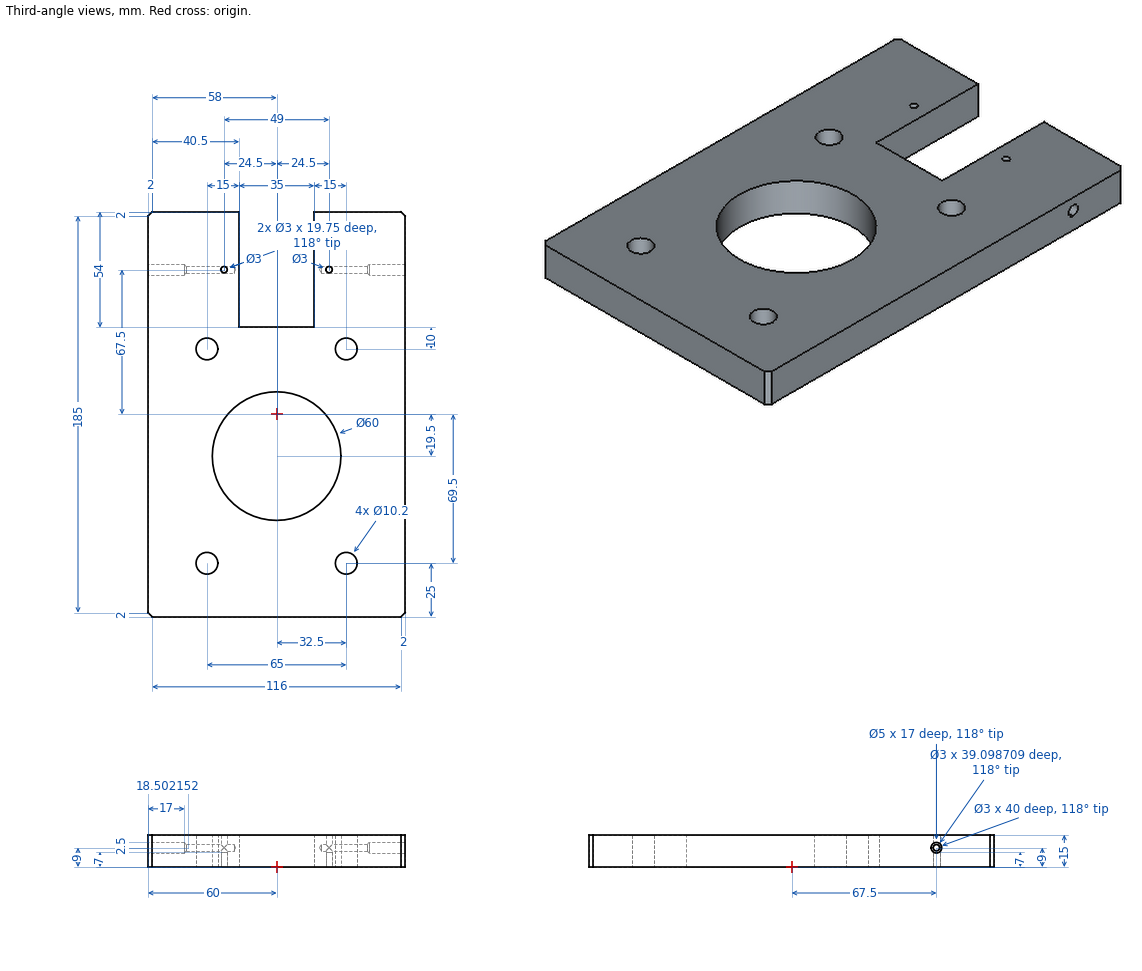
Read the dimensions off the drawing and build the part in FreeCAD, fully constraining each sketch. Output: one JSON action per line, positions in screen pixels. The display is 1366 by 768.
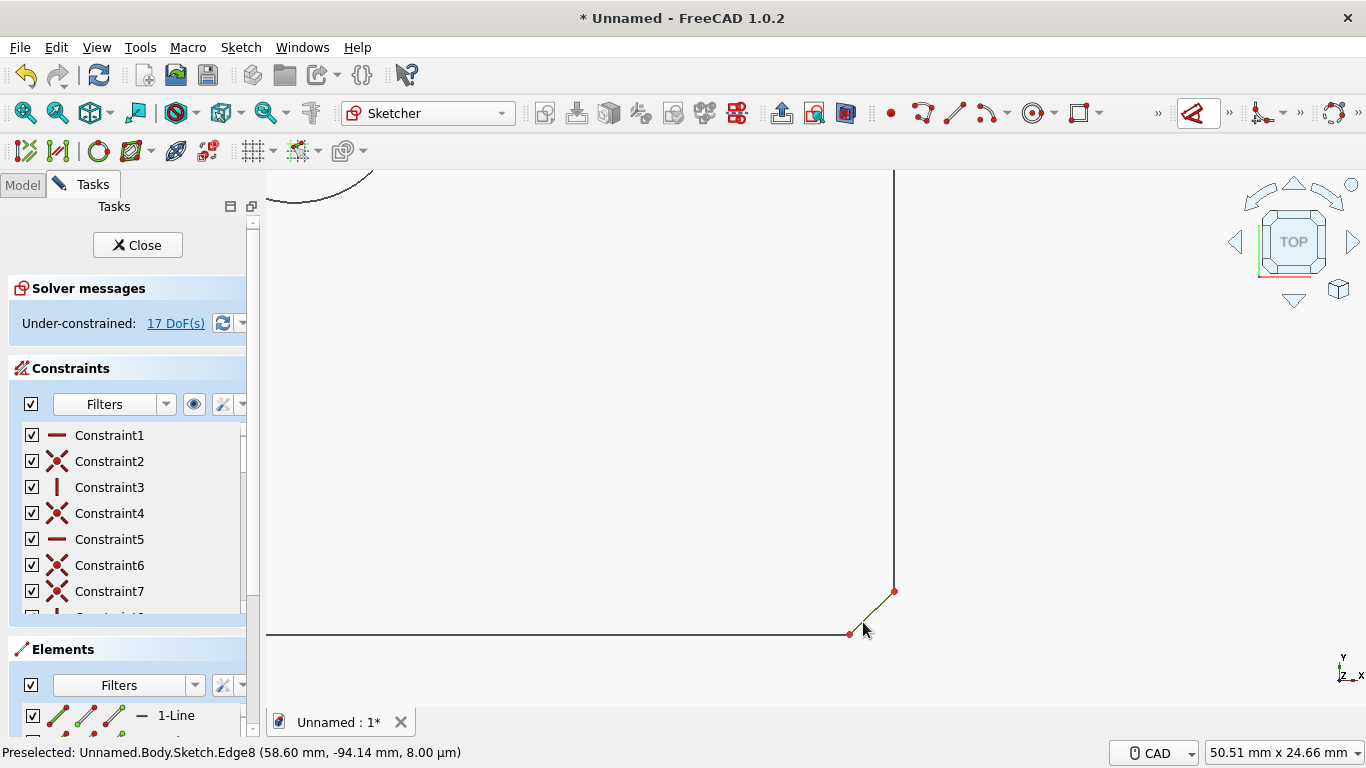
{"action": "key", "text": "l"}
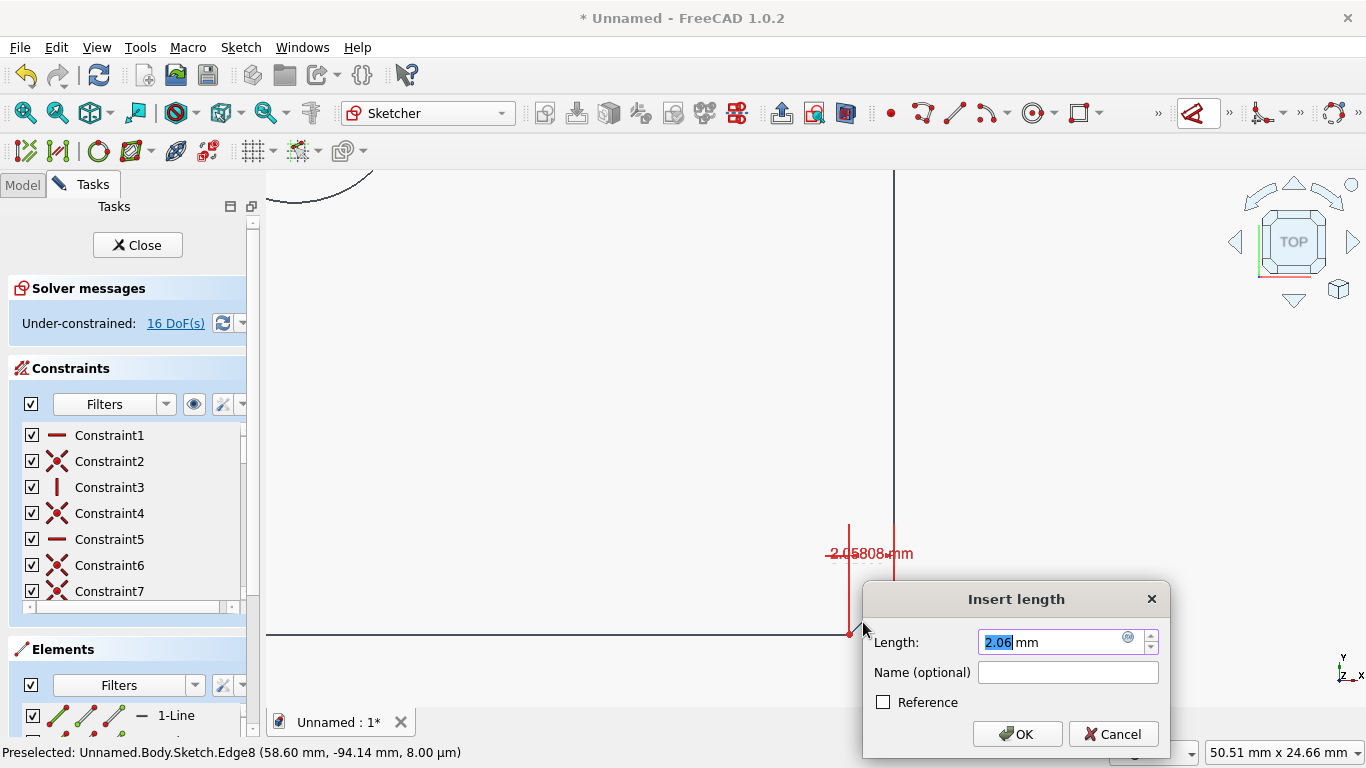
{"action": "type", "text": "2"}
{"action": "key", "text": "Return"}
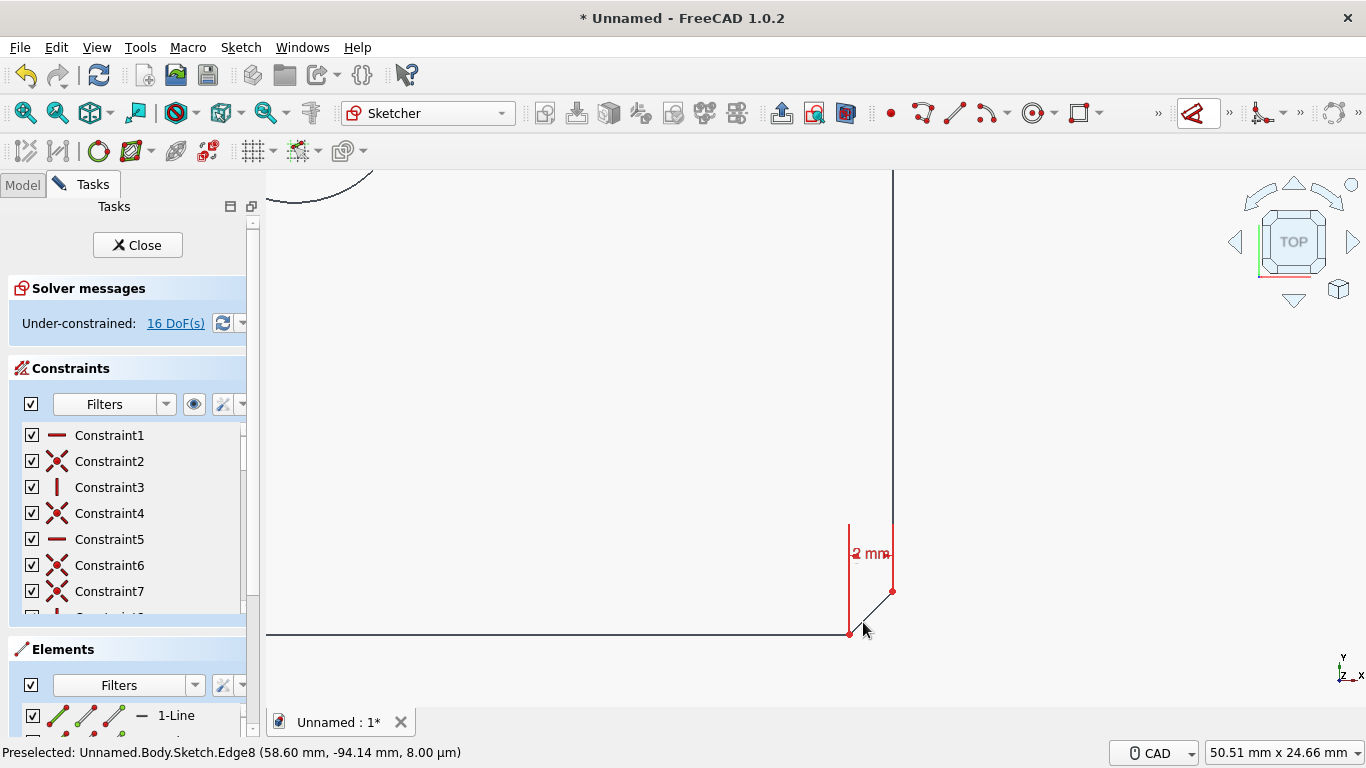
{"action": "left_click", "coordinate": [862, 622]}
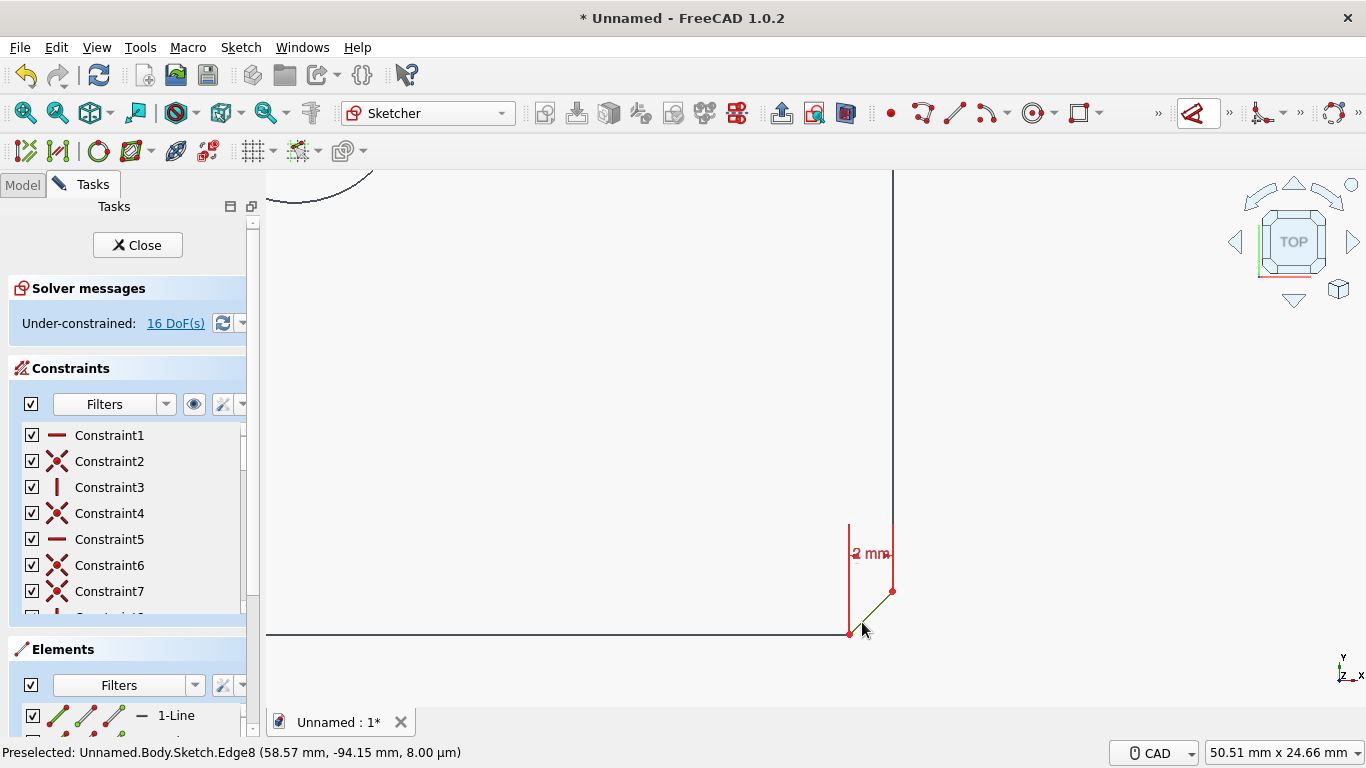
{"action": "key", "text": "i"}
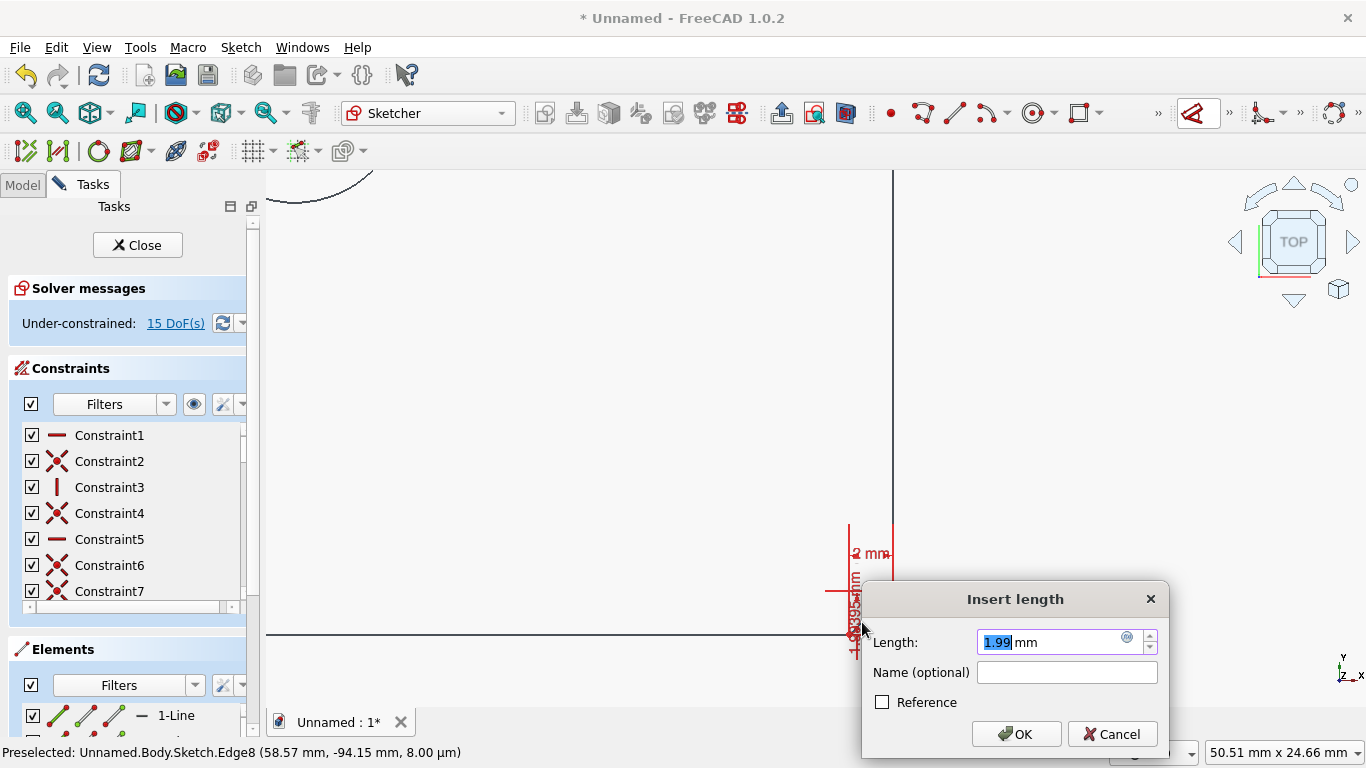
{"action": "type", "text": "2"}
{"action": "key", "text": "Return"}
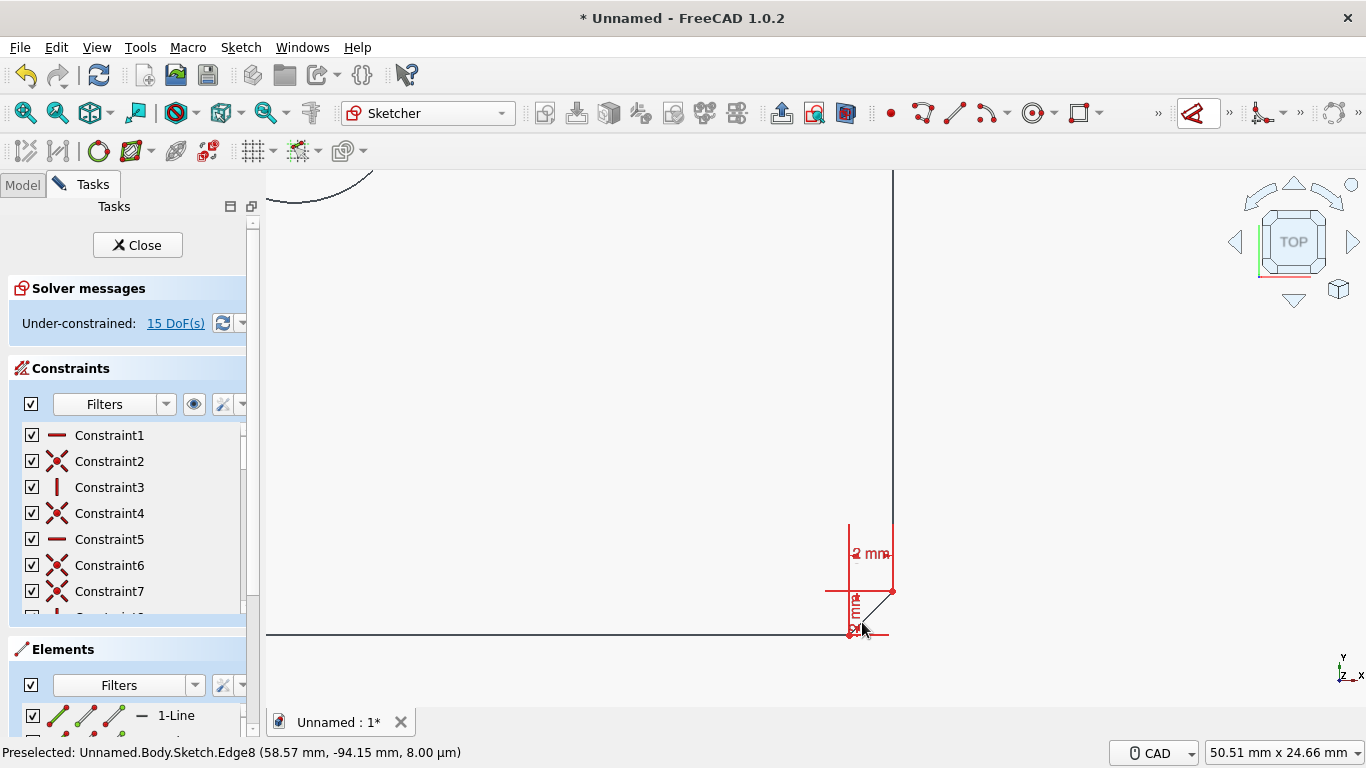
{"action": "scroll", "coordinate": [863, 625], "scroll_direction": "down", "scroll_amount": 12}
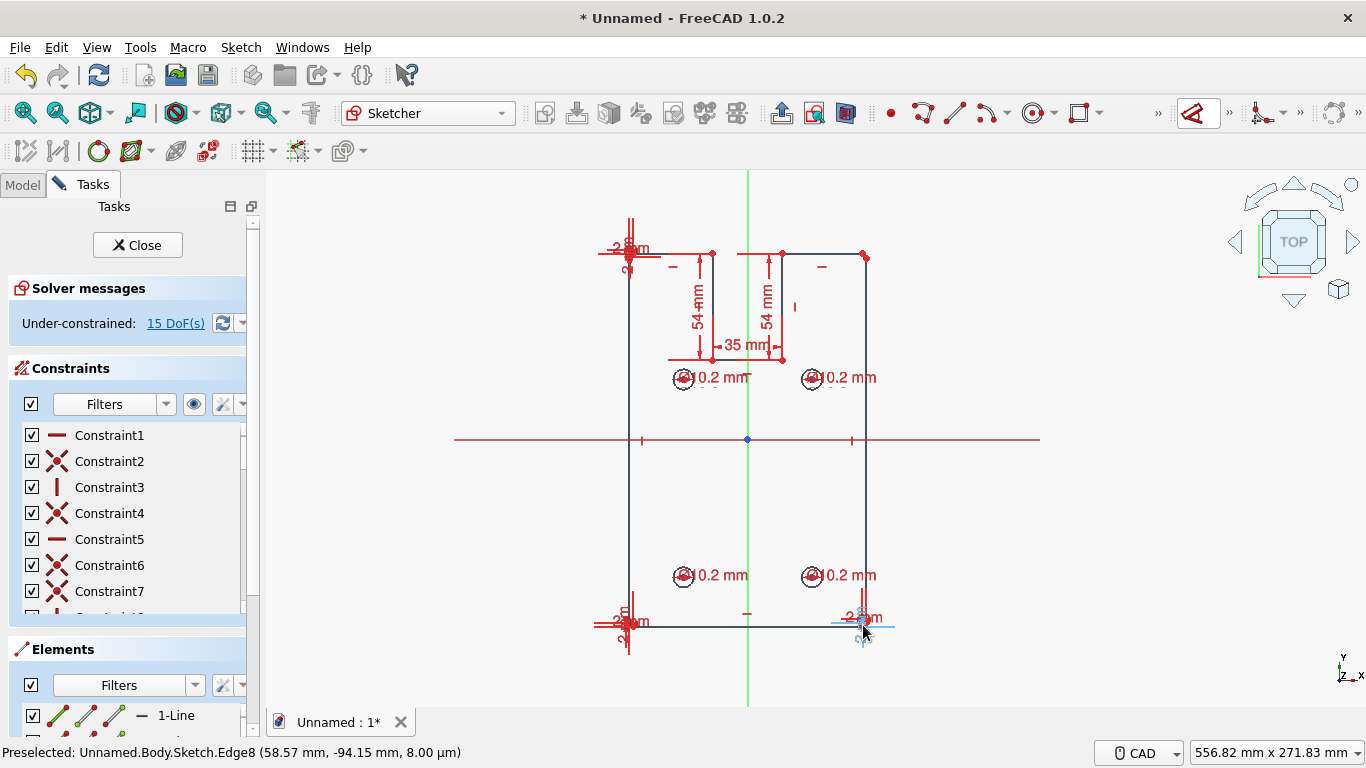
{"action": "scroll", "coordinate": [865, 257], "scroll_direction": "up", "scroll_amount": 12}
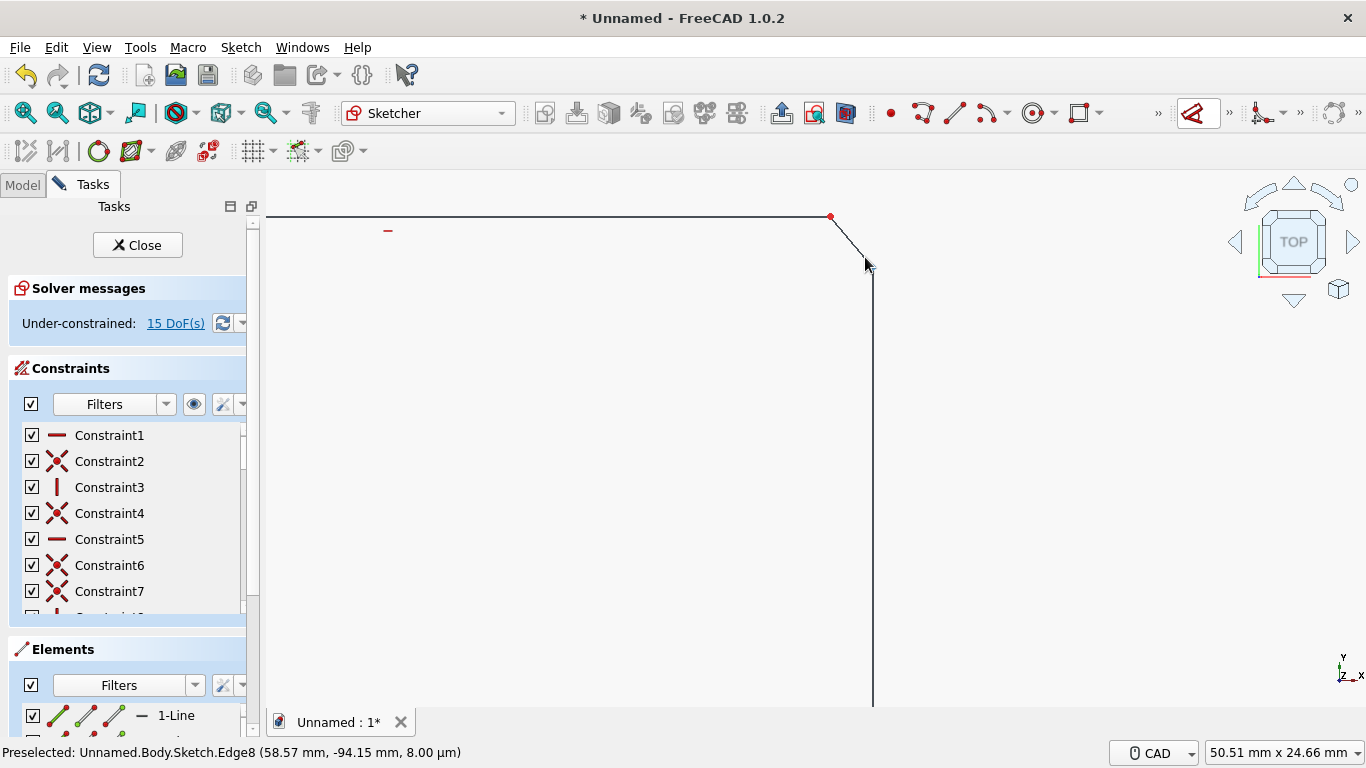
{"action": "left_click", "coordinate": [860, 252]}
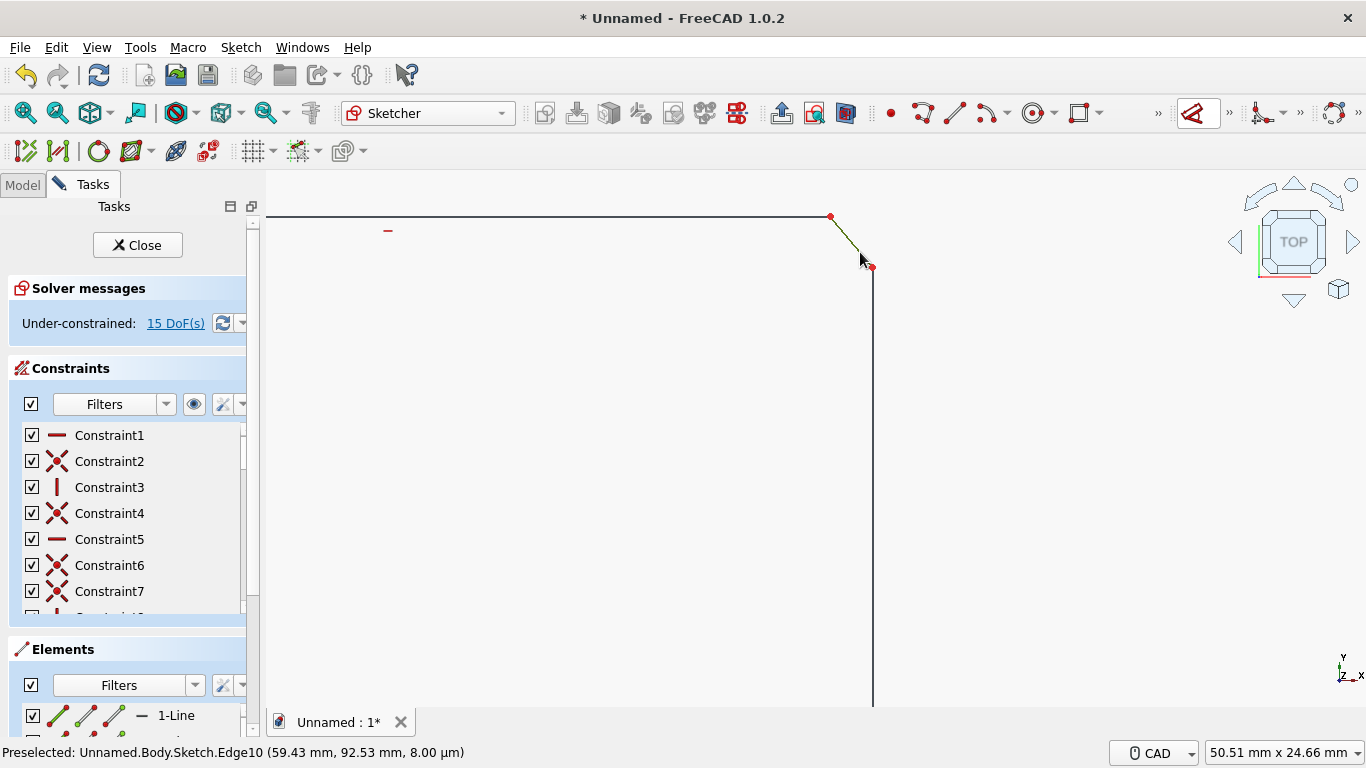
{"action": "left_click", "coordinate": [1214, 114]}